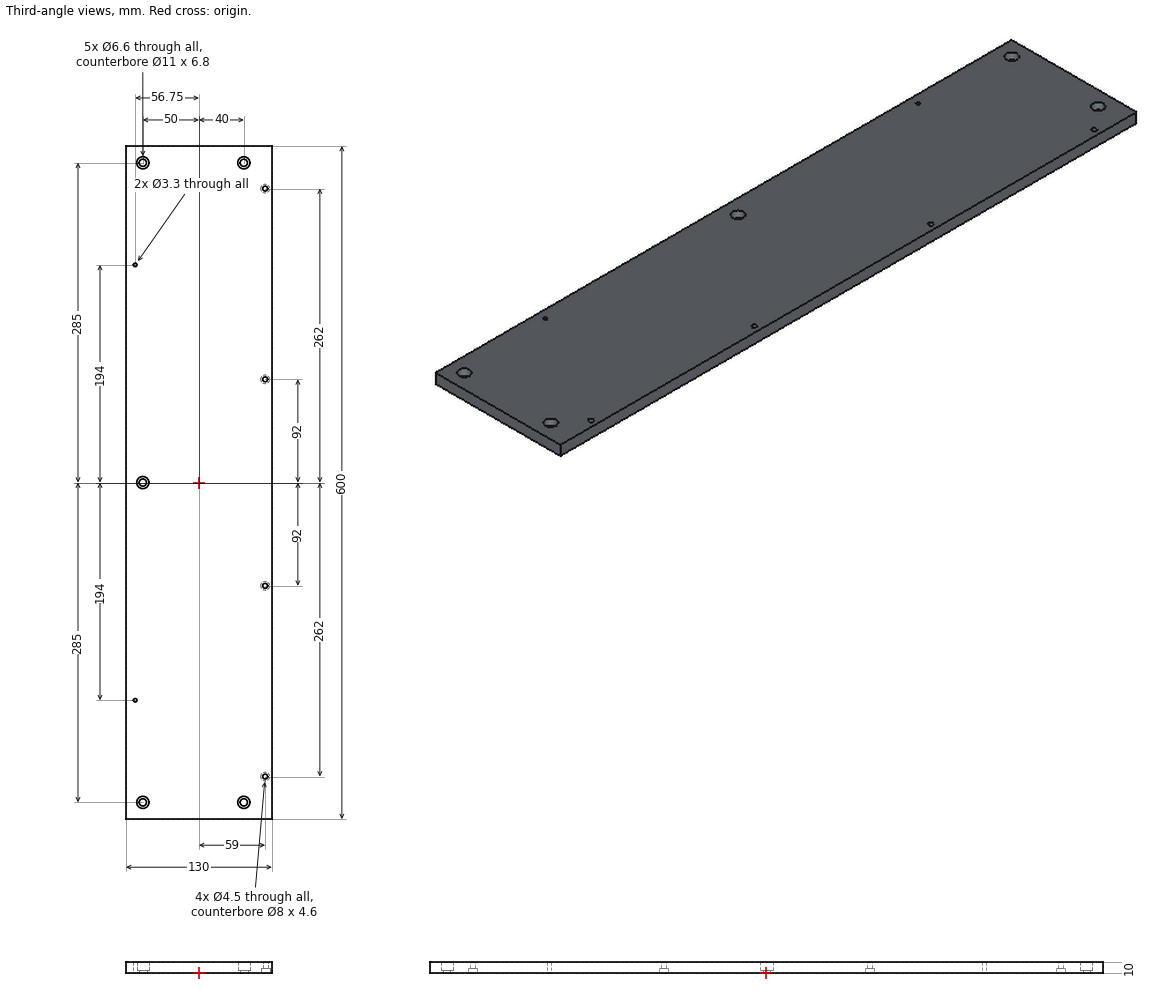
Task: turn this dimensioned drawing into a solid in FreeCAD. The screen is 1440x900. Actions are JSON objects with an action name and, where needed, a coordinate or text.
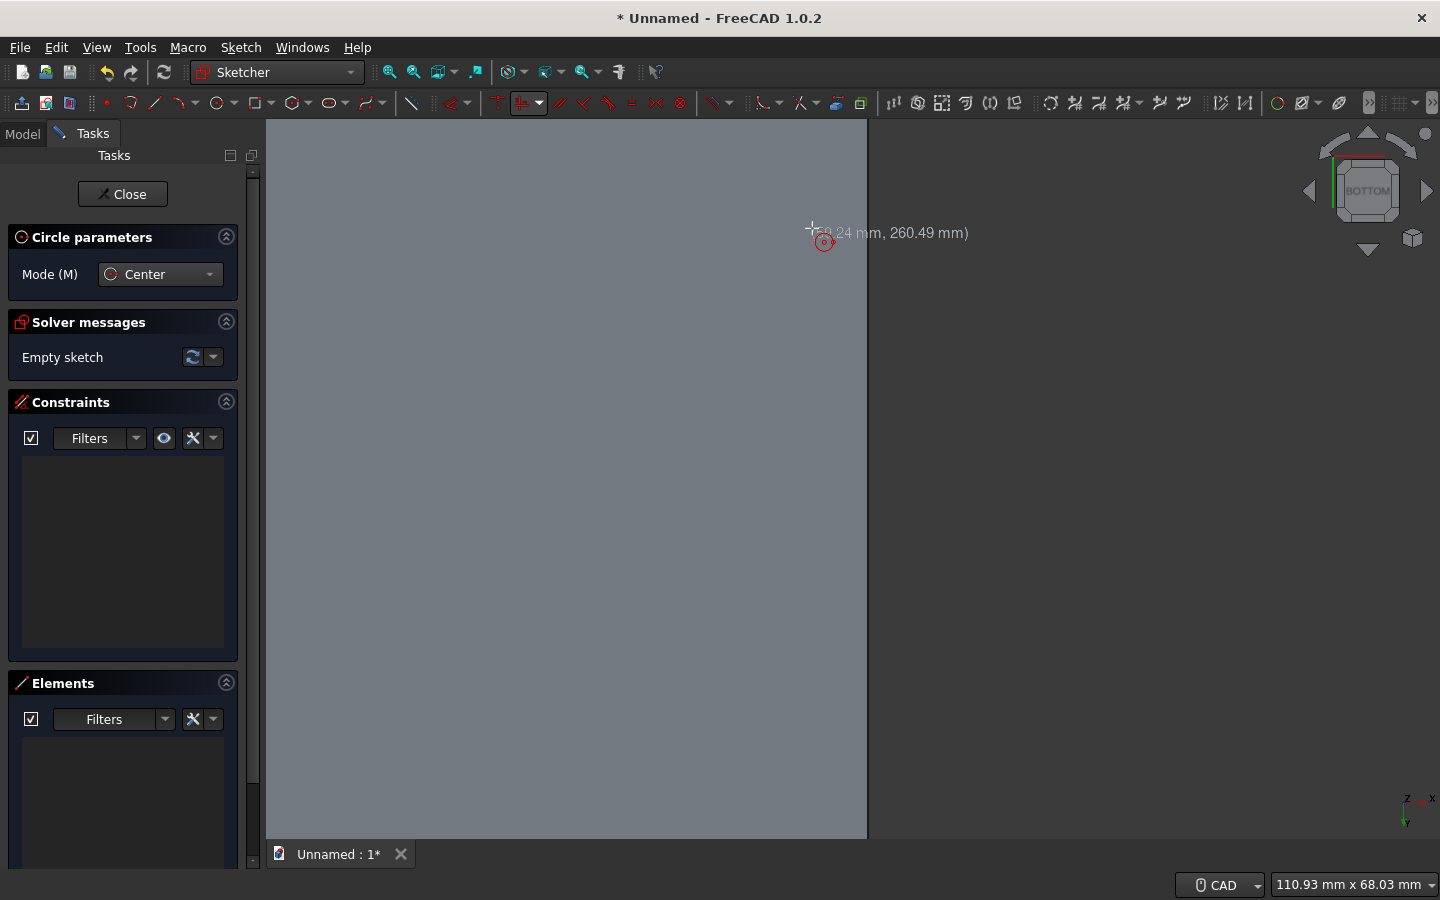
{"action": "scroll", "coordinate": [812, 228], "scroll_direction": "down", "scroll_amount": 12}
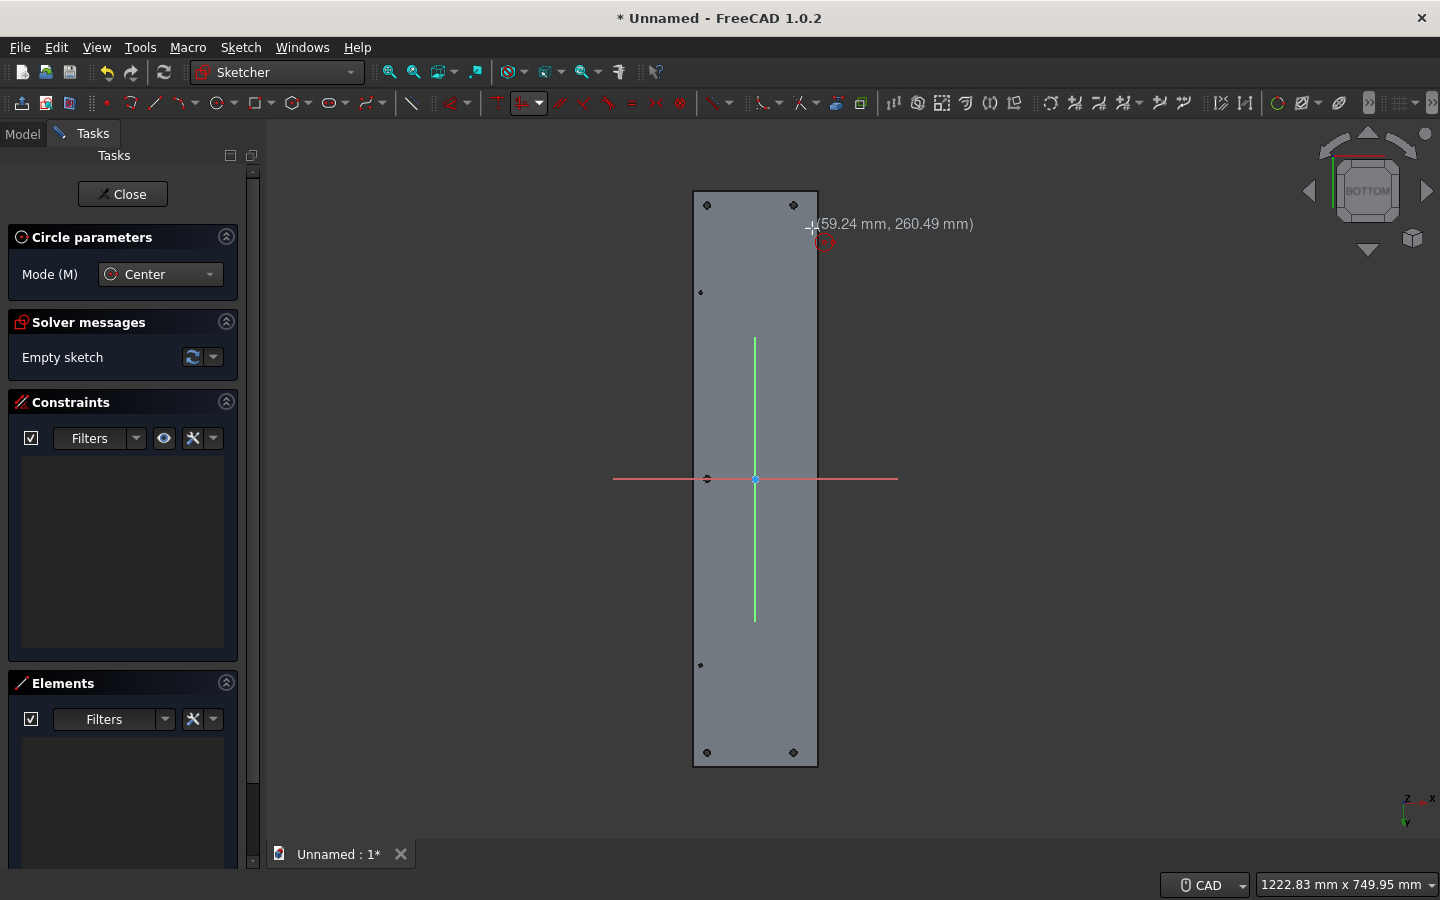
{"action": "left_click", "coordinate": [812, 228]}
{"action": "mouse_move", "coordinate": [813, 226]}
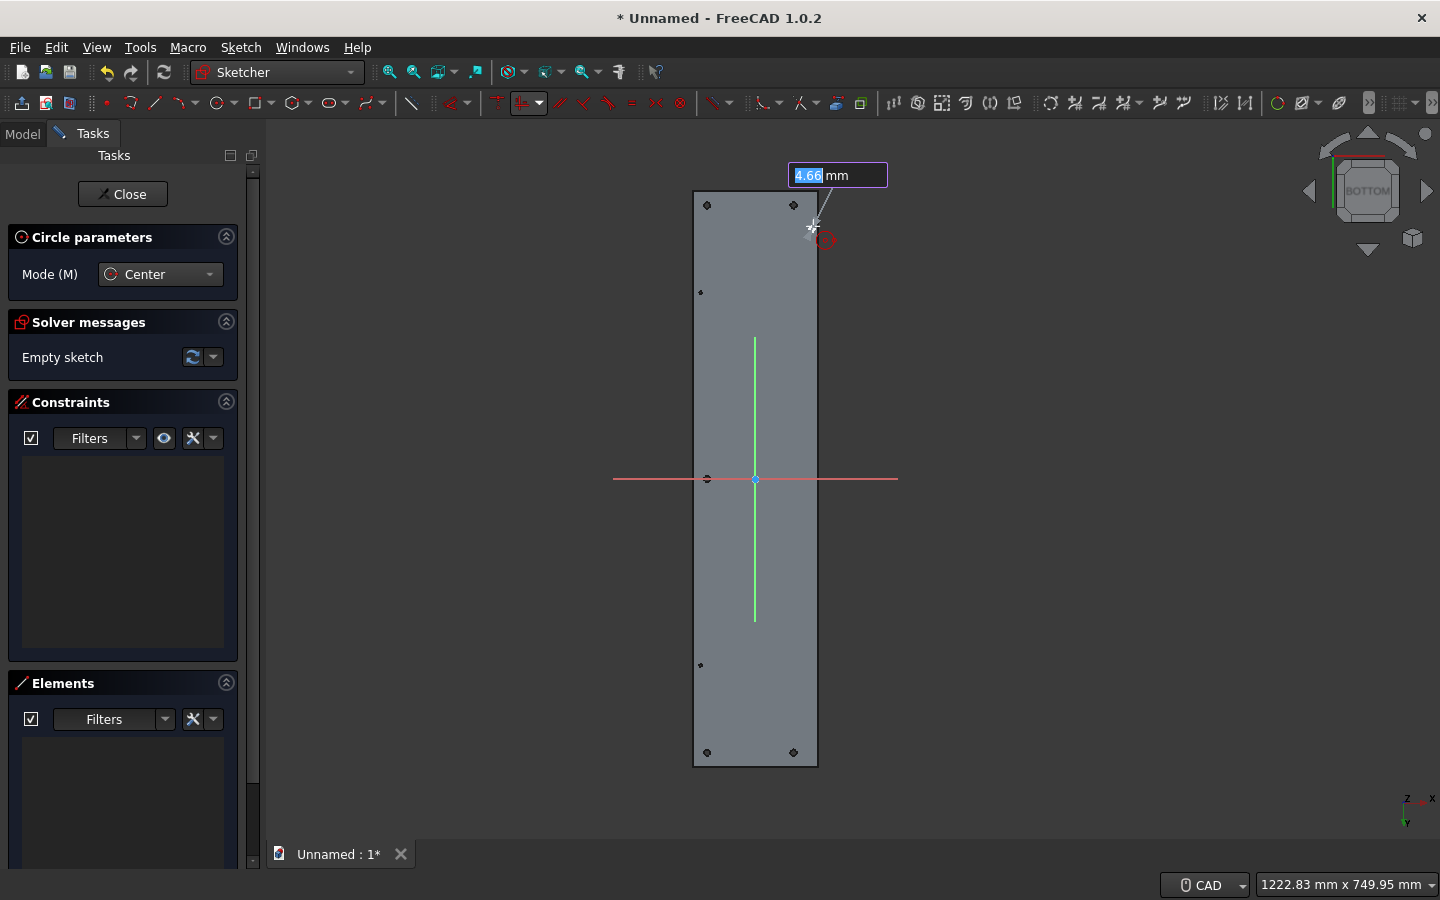
{"action": "type", "text": "4.5"}
{"action": "key", "text": "Return"}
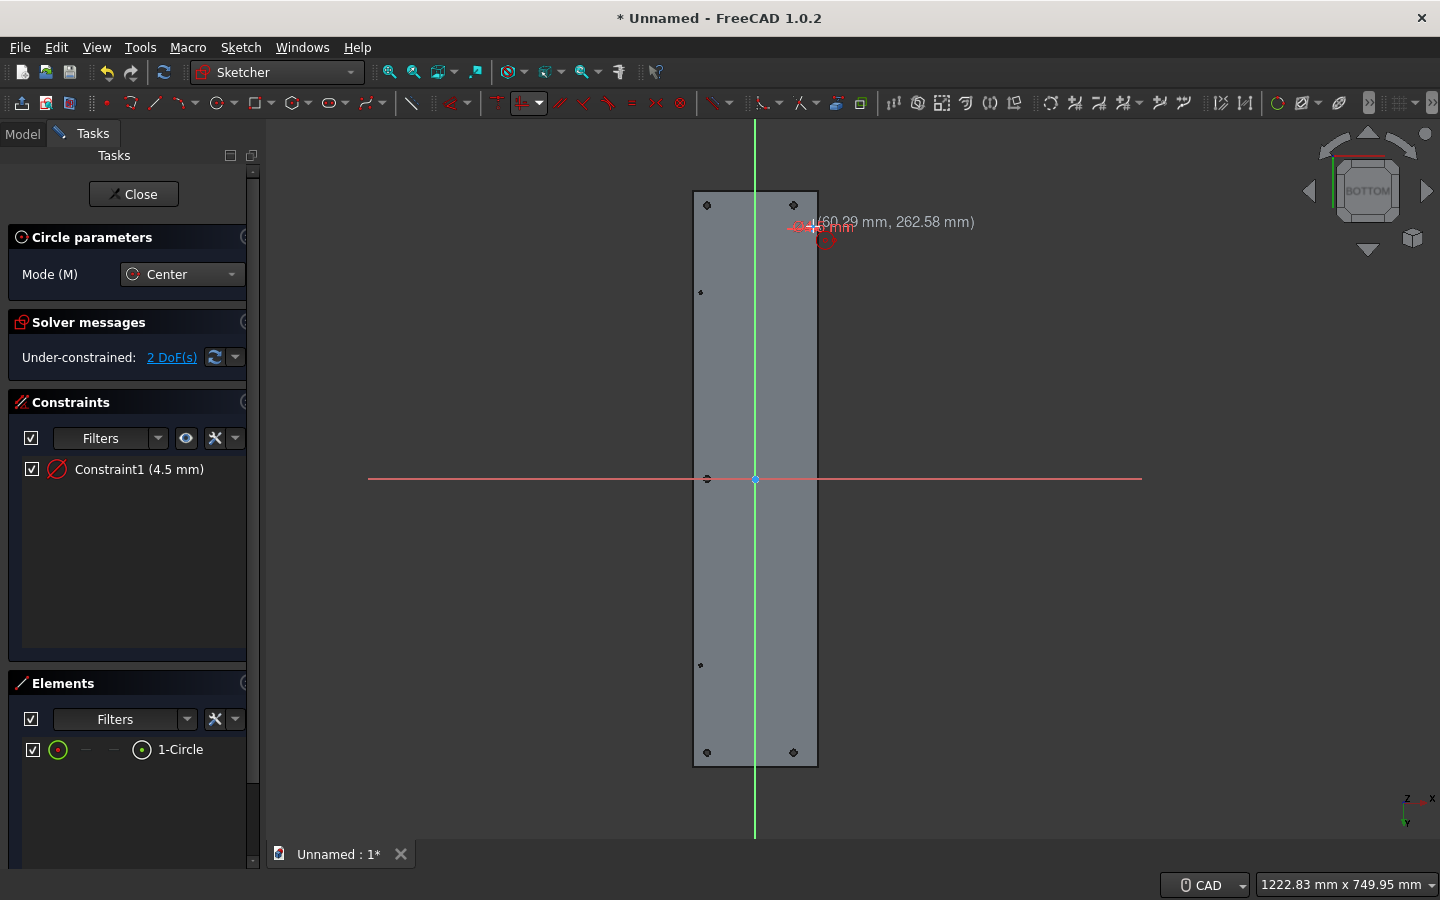
{"action": "scroll", "coordinate": [812, 391], "scroll_direction": "up", "scroll_amount": 12}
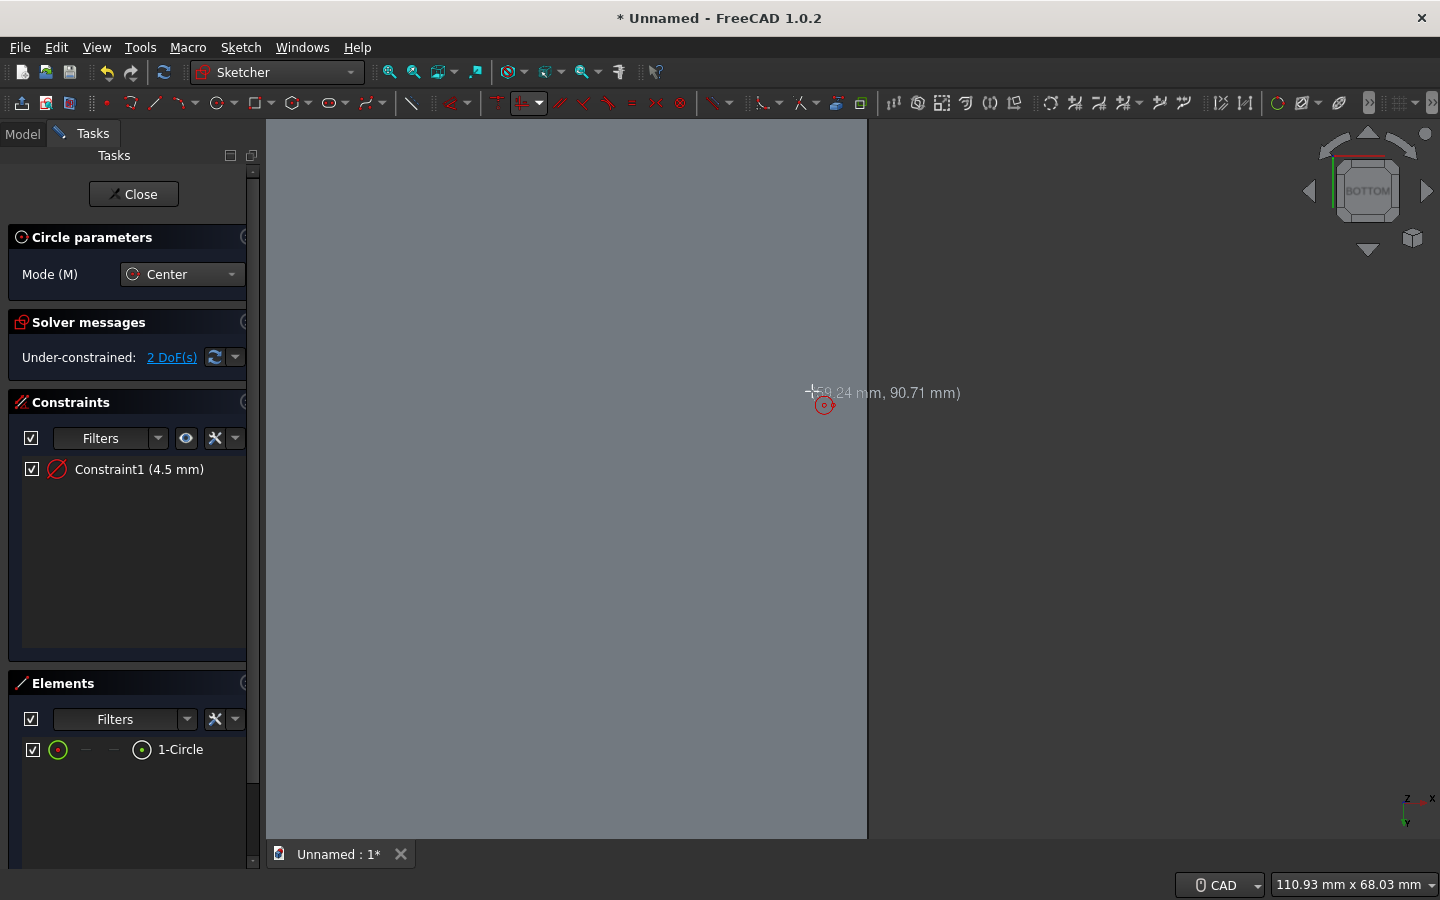
{"action": "scroll", "coordinate": [812, 391], "scroll_direction": "down", "scroll_amount": 12}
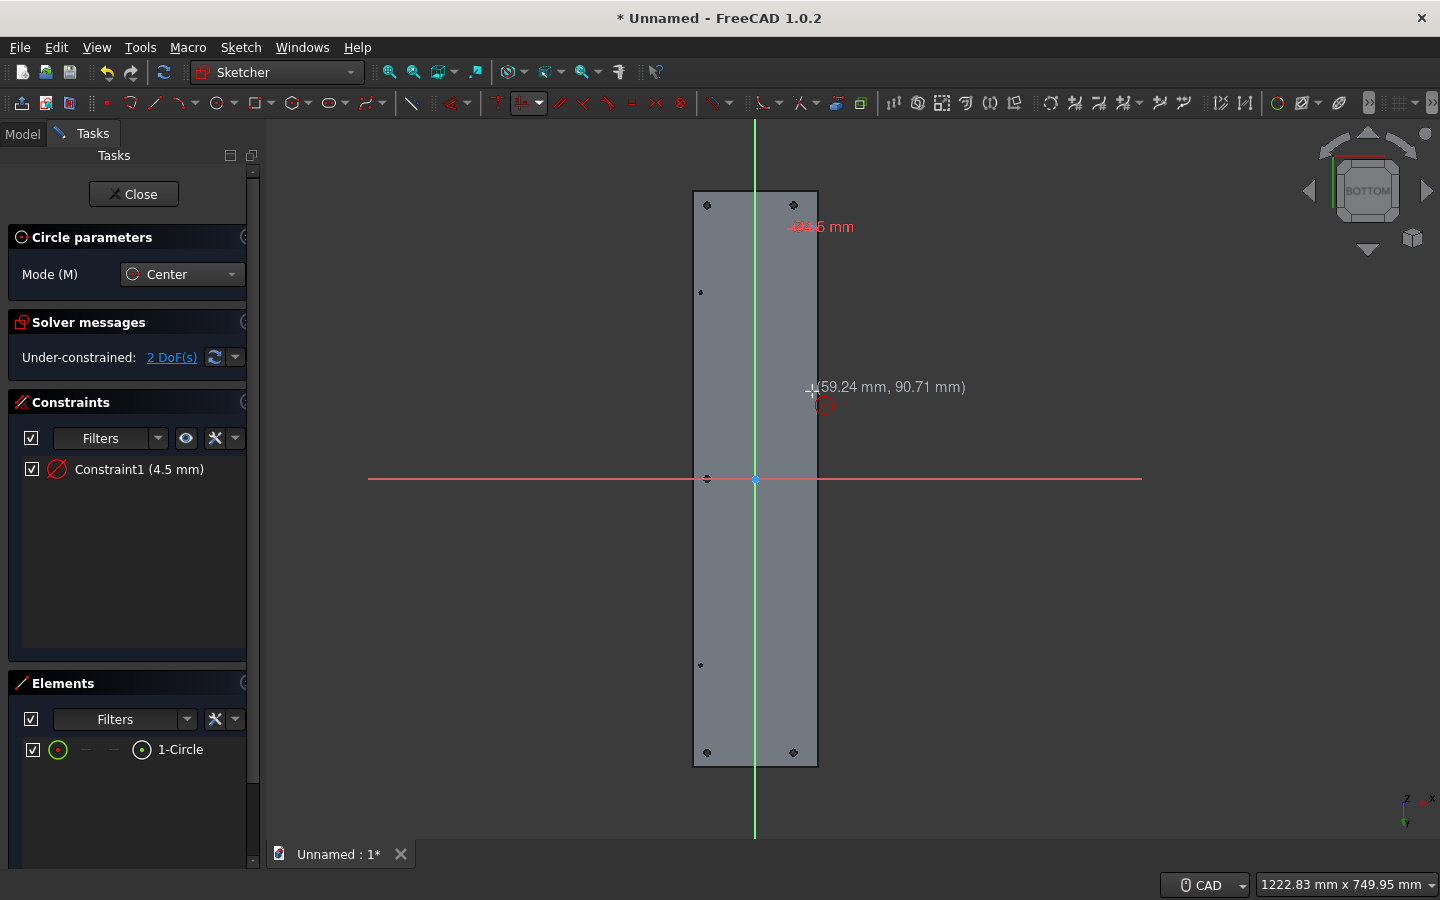
{"action": "left_click", "coordinate": [812, 391]}
{"action": "mouse_move", "coordinate": [813, 389]}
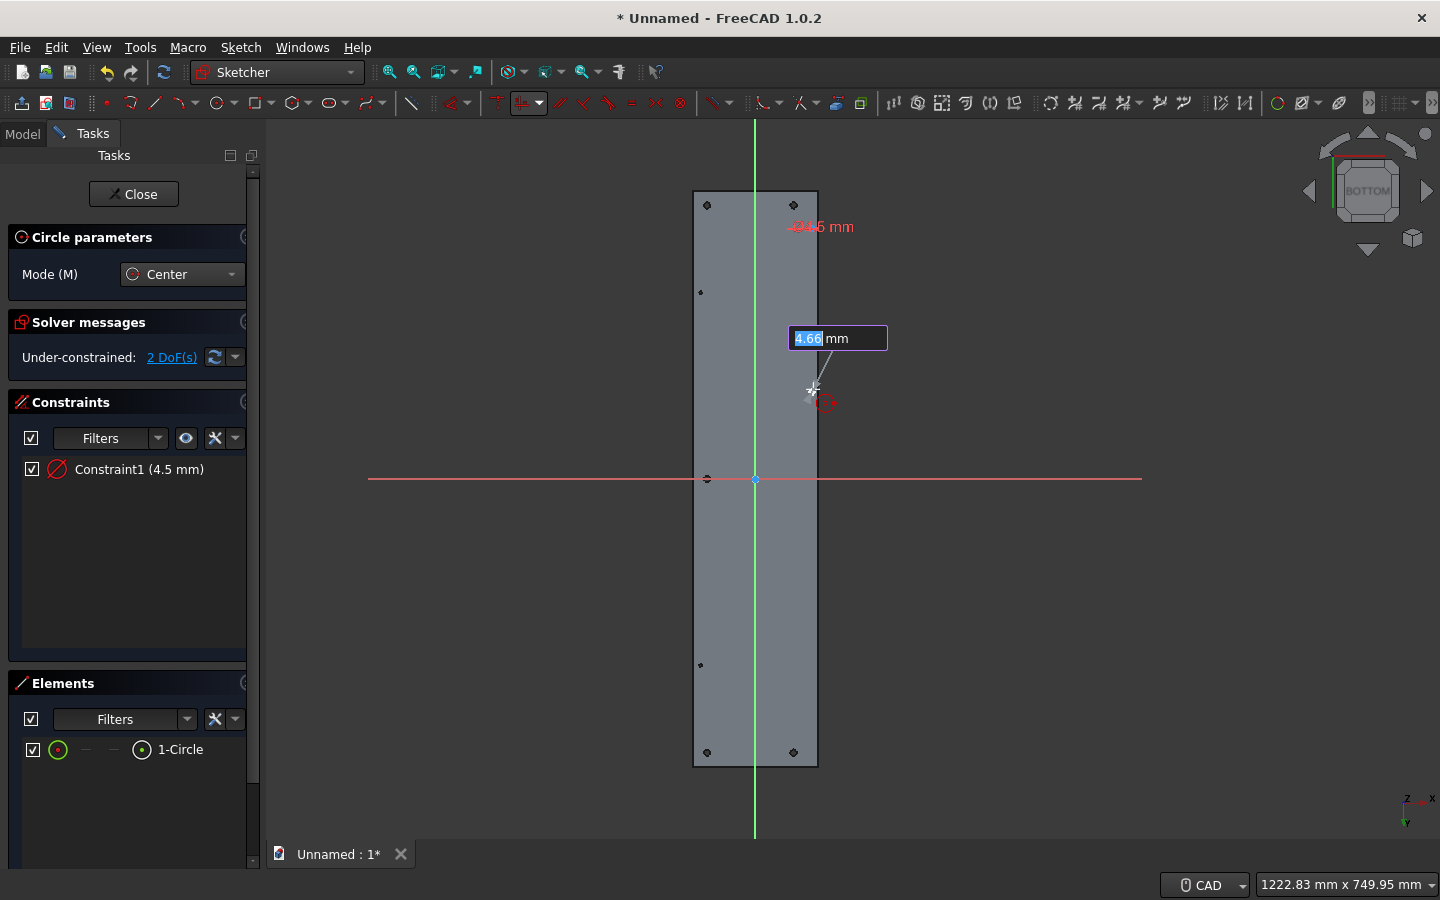
{"action": "type", "text": "4.5"}
{"action": "key", "text": "Return"}